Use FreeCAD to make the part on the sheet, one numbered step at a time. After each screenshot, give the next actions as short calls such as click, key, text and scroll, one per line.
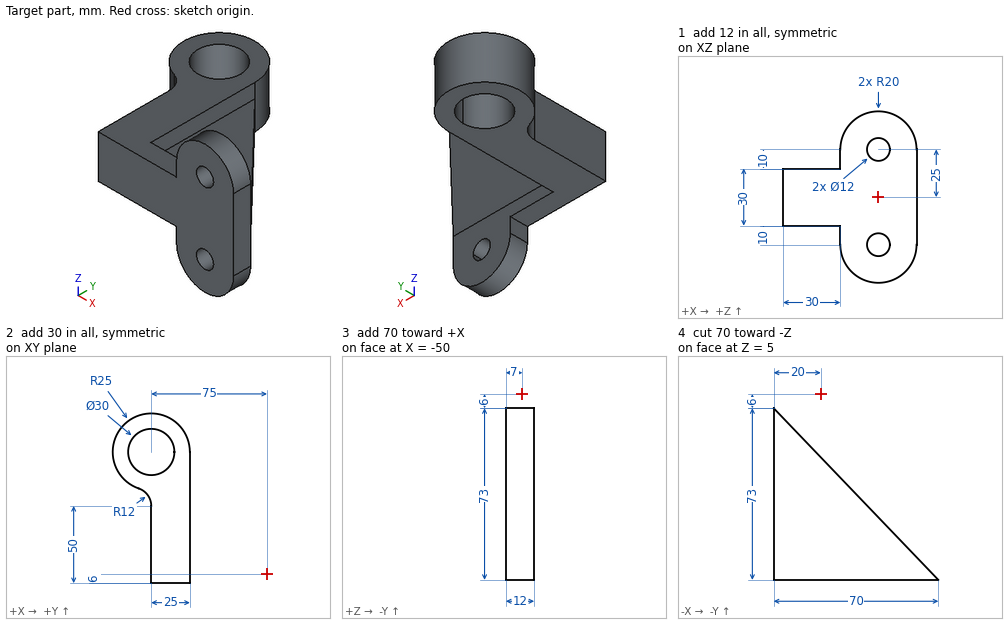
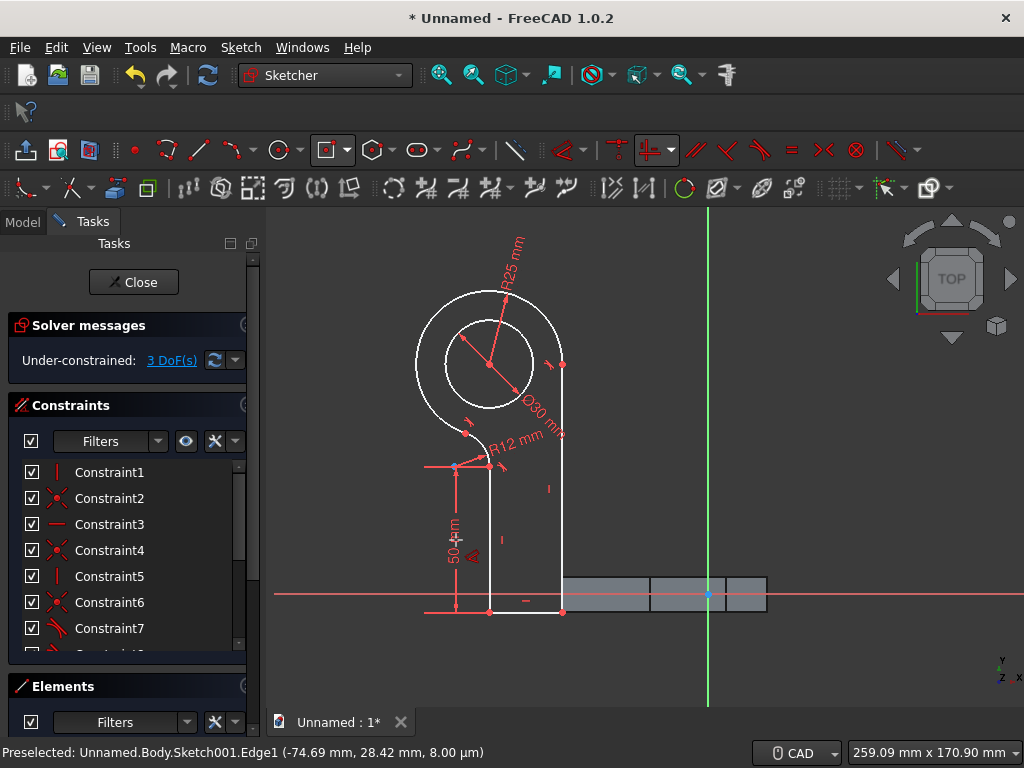
click(512, 613)
click(526, 647)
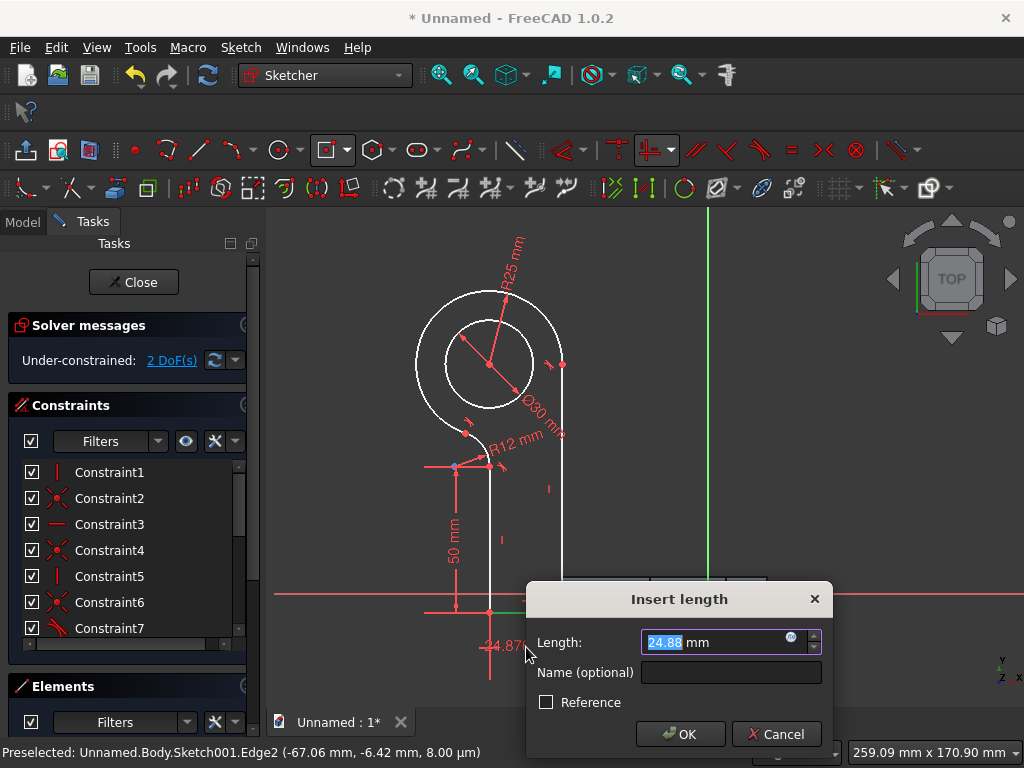
text(25)
key(Return)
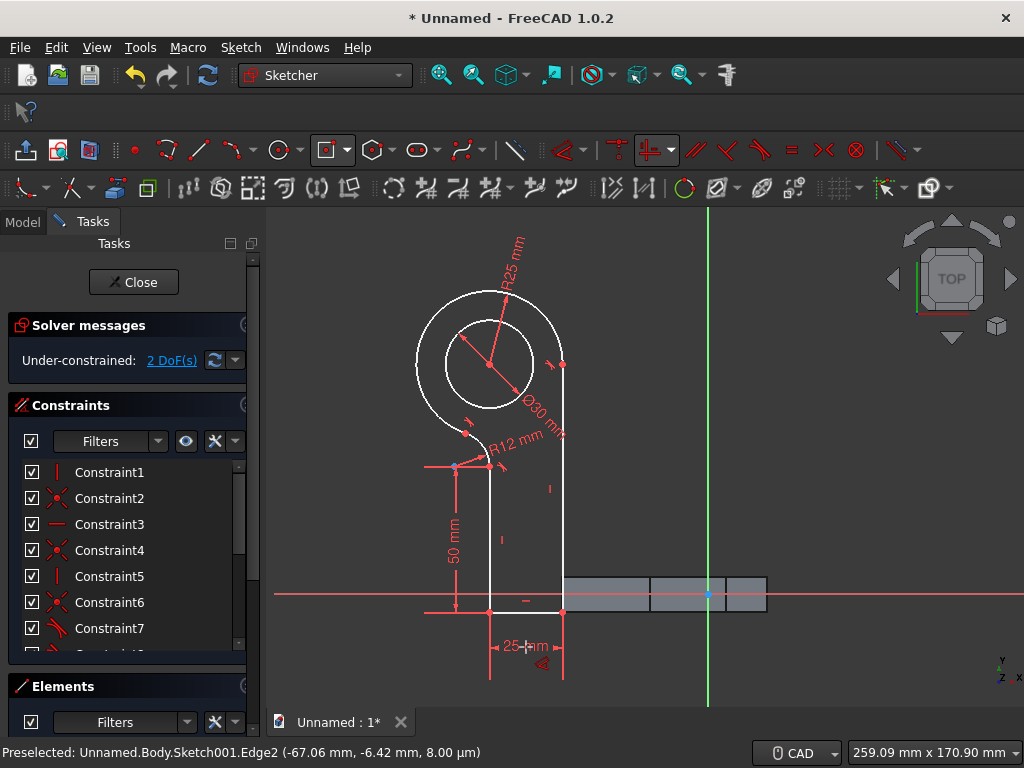
scroll(490, 613, up, 5)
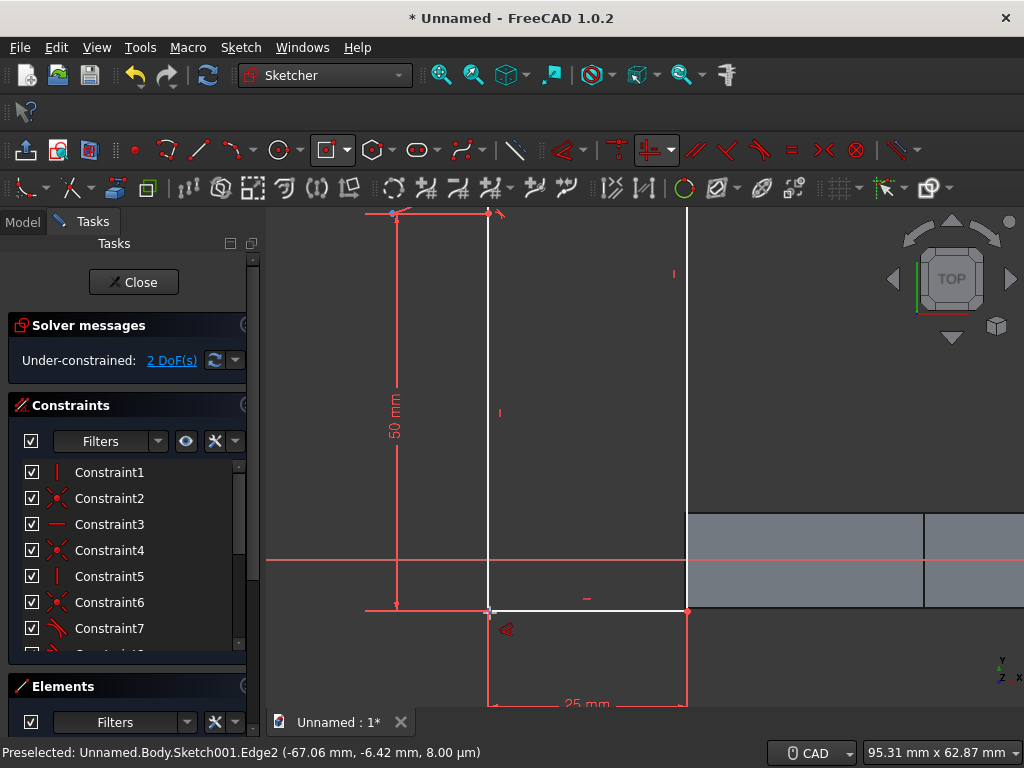
click(488, 611)
click(454, 586)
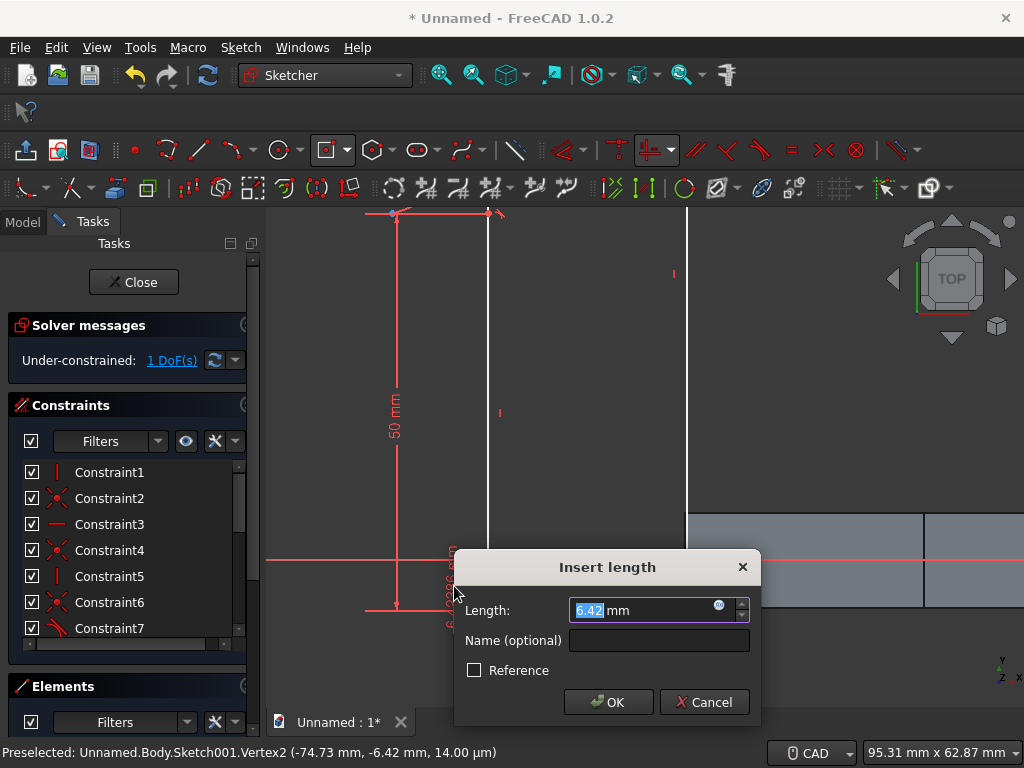
text(6)
key(Return)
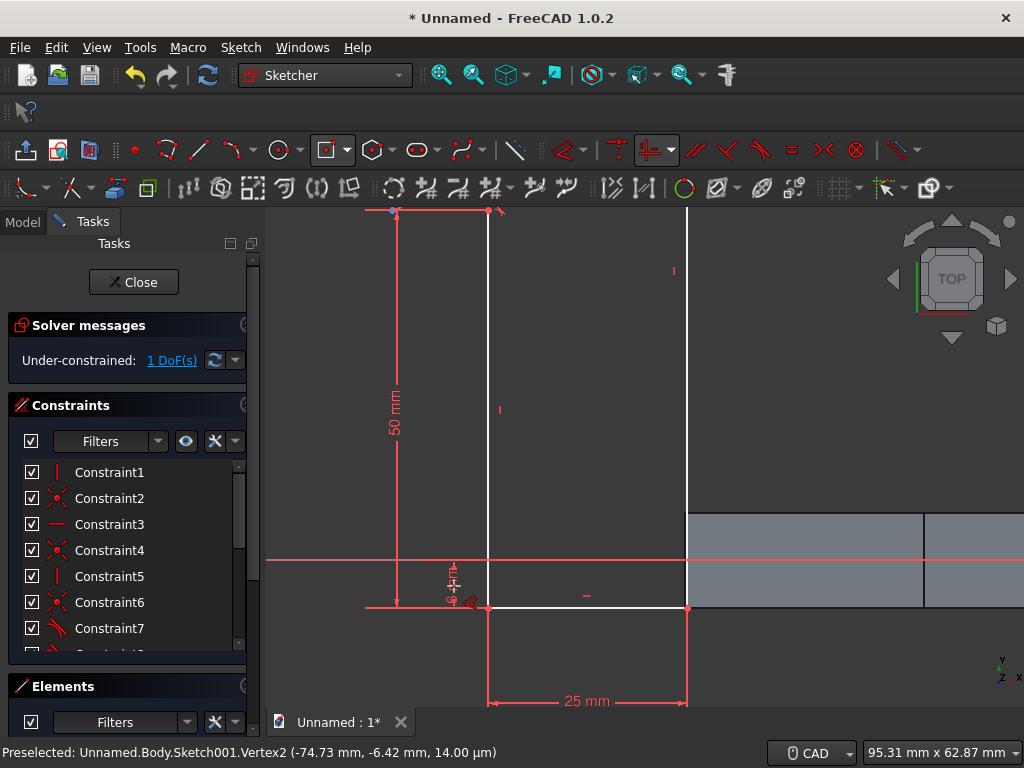
scroll(490, 613, down, 5)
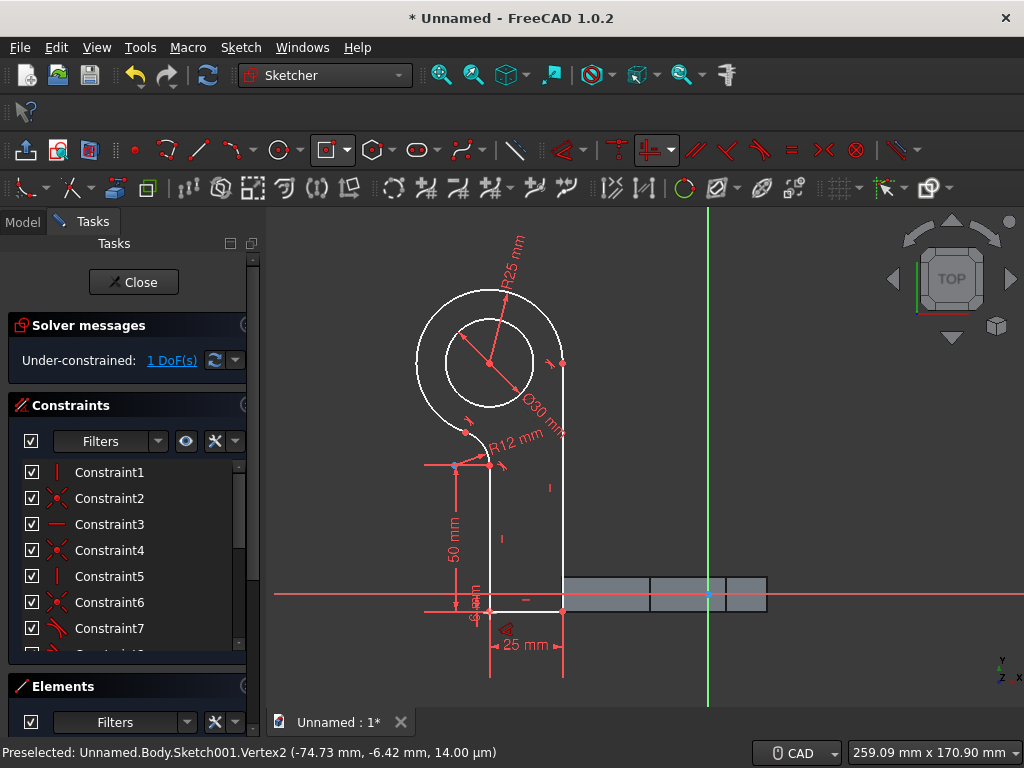
click(490, 363)
click(599, 628)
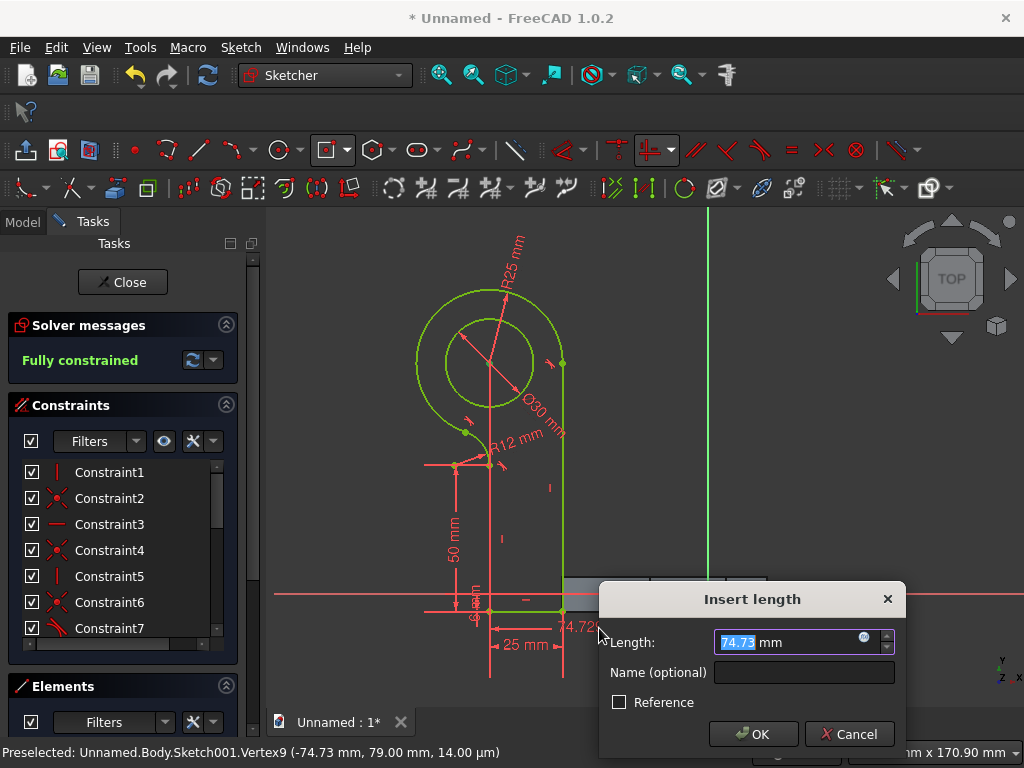
text(75)
key(Return)
key(Escape)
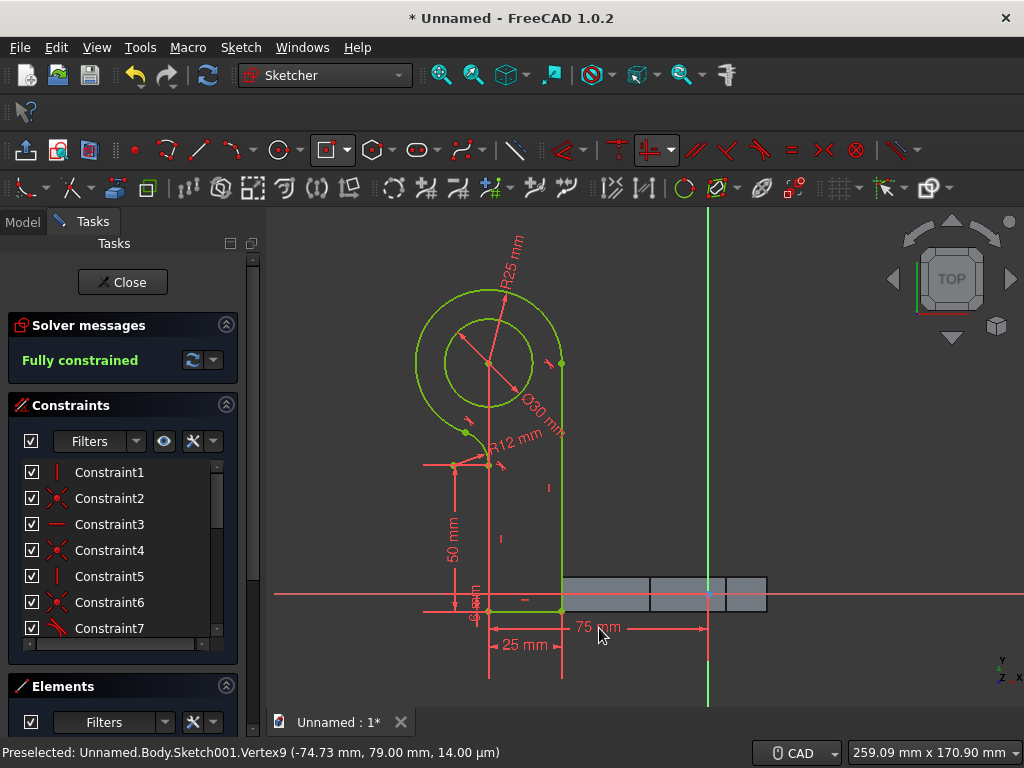
click(123, 282)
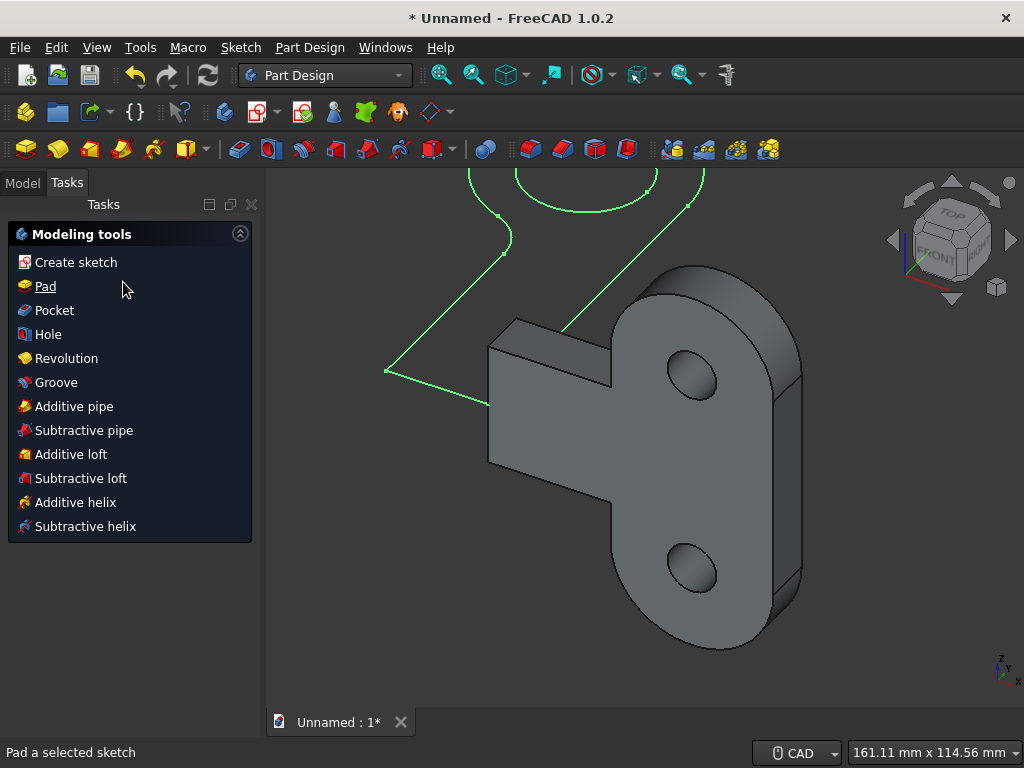
click(26, 150)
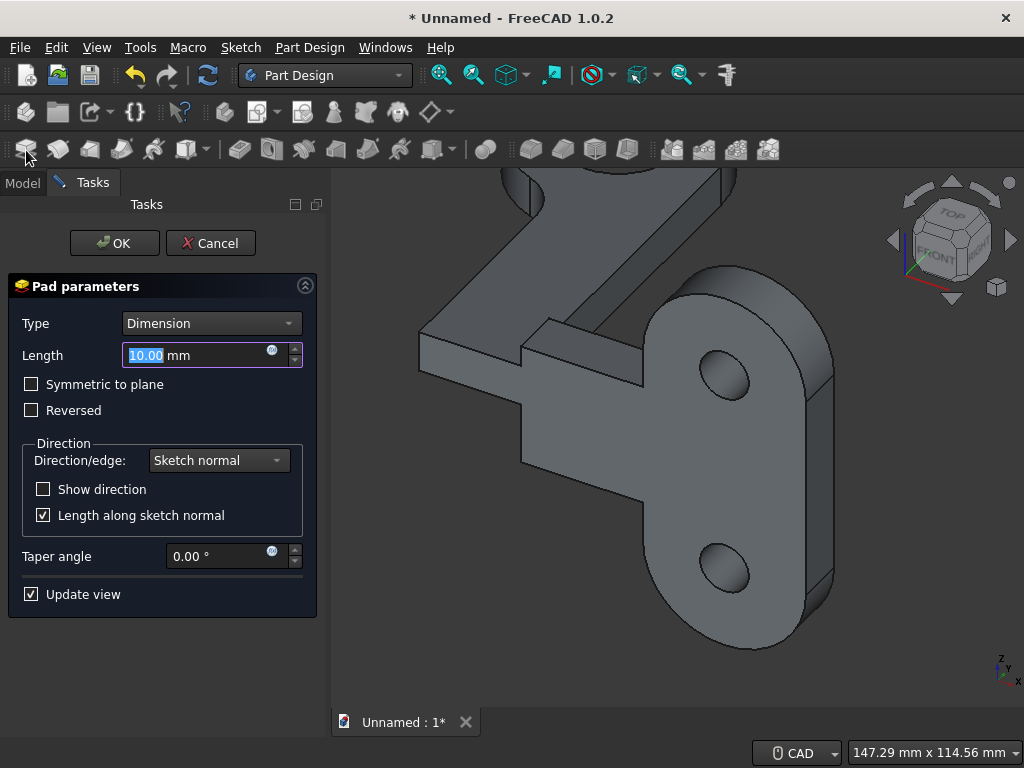
text(30)
key(Tab)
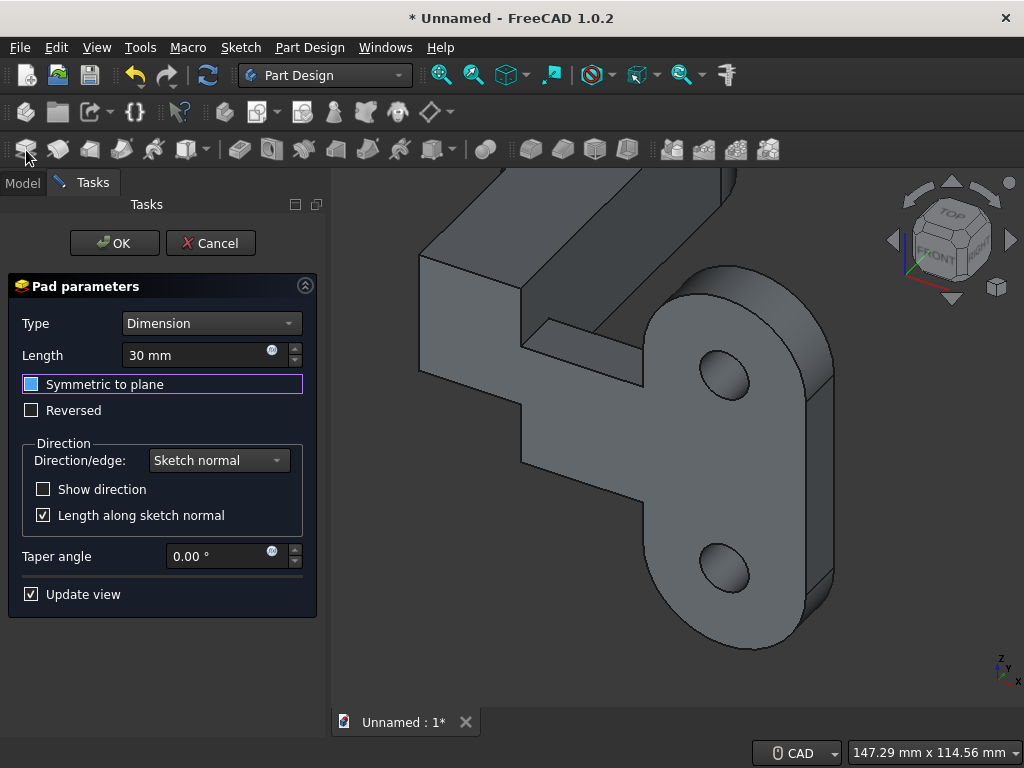
click(30, 384)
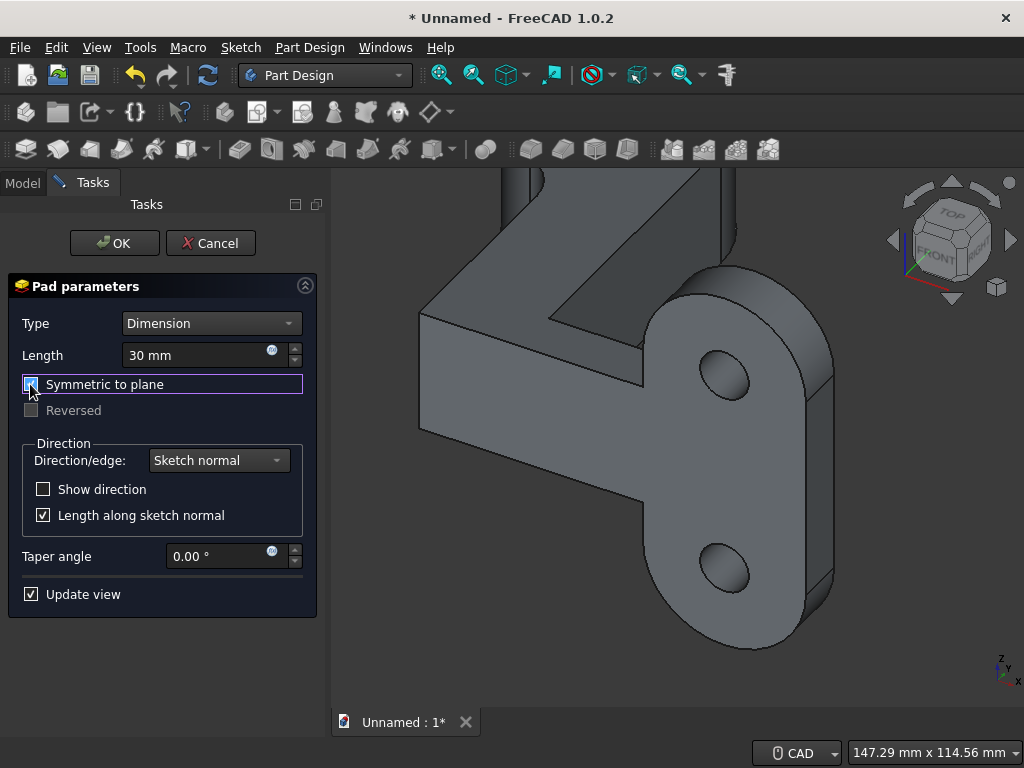
click(115, 243)